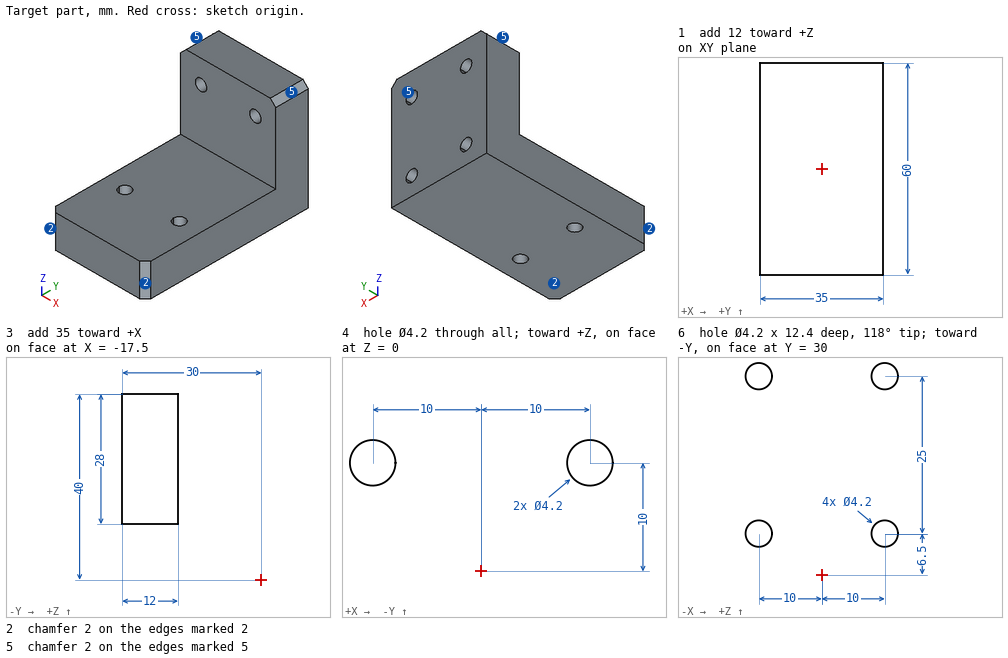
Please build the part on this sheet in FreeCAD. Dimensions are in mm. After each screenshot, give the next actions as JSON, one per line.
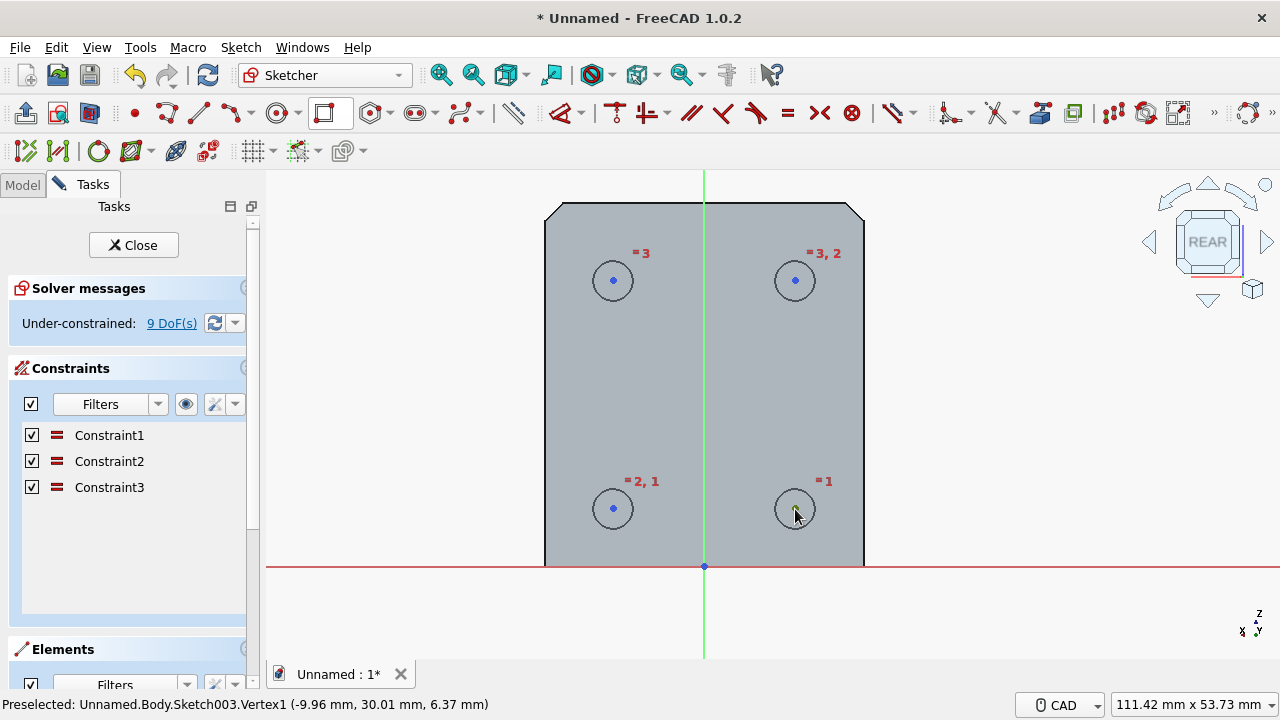
{"action": "left_click", "coordinate": [613, 509]}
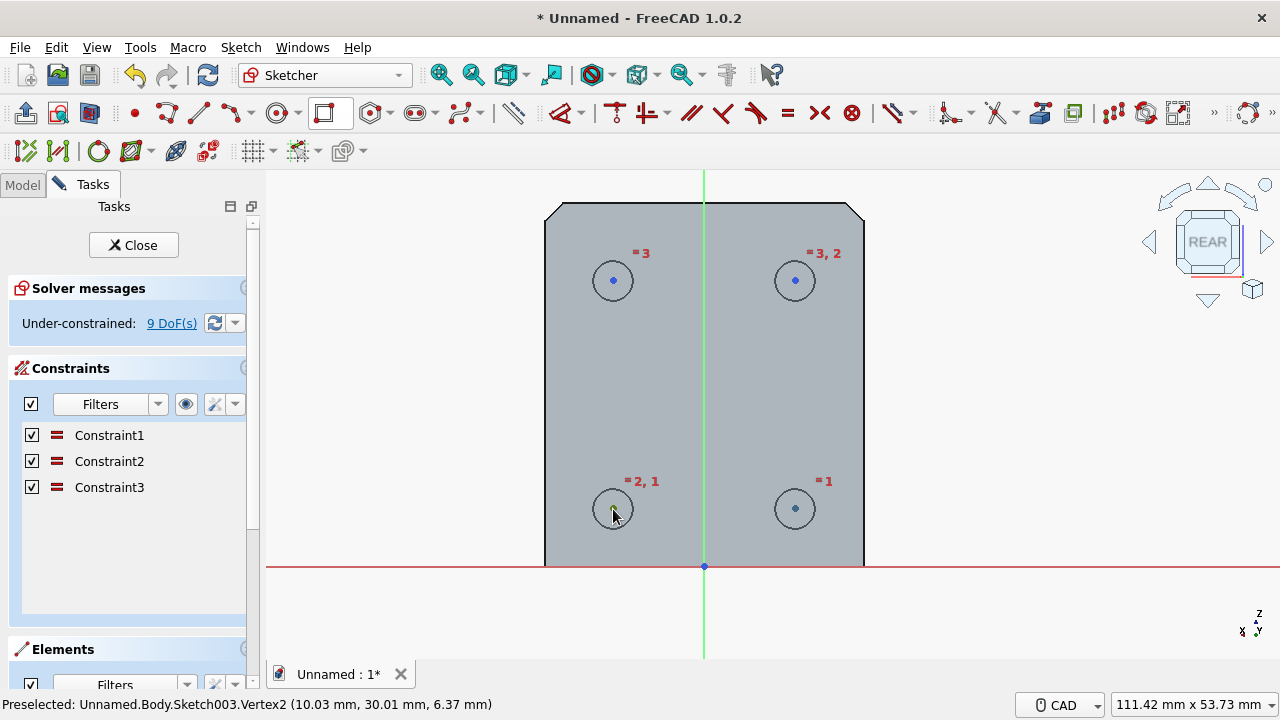
{"action": "left_click", "coordinate": [670, 114]}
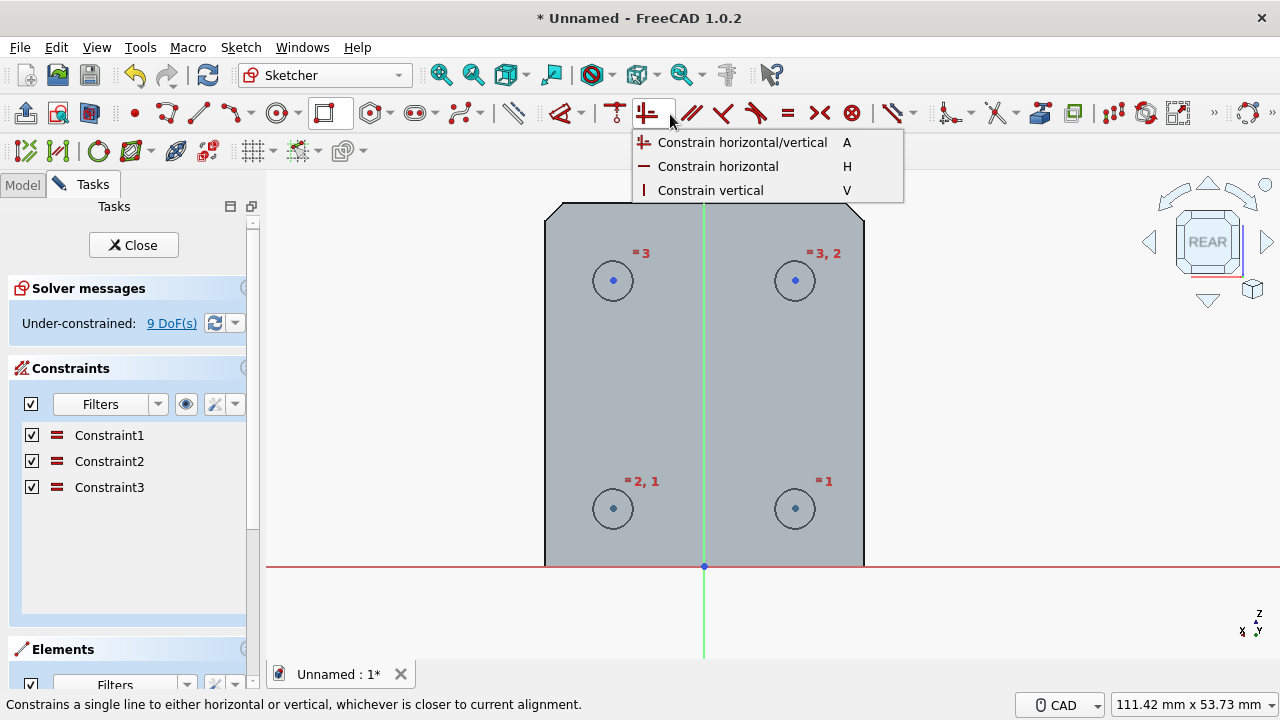
{"action": "left_click", "coordinate": [768, 166]}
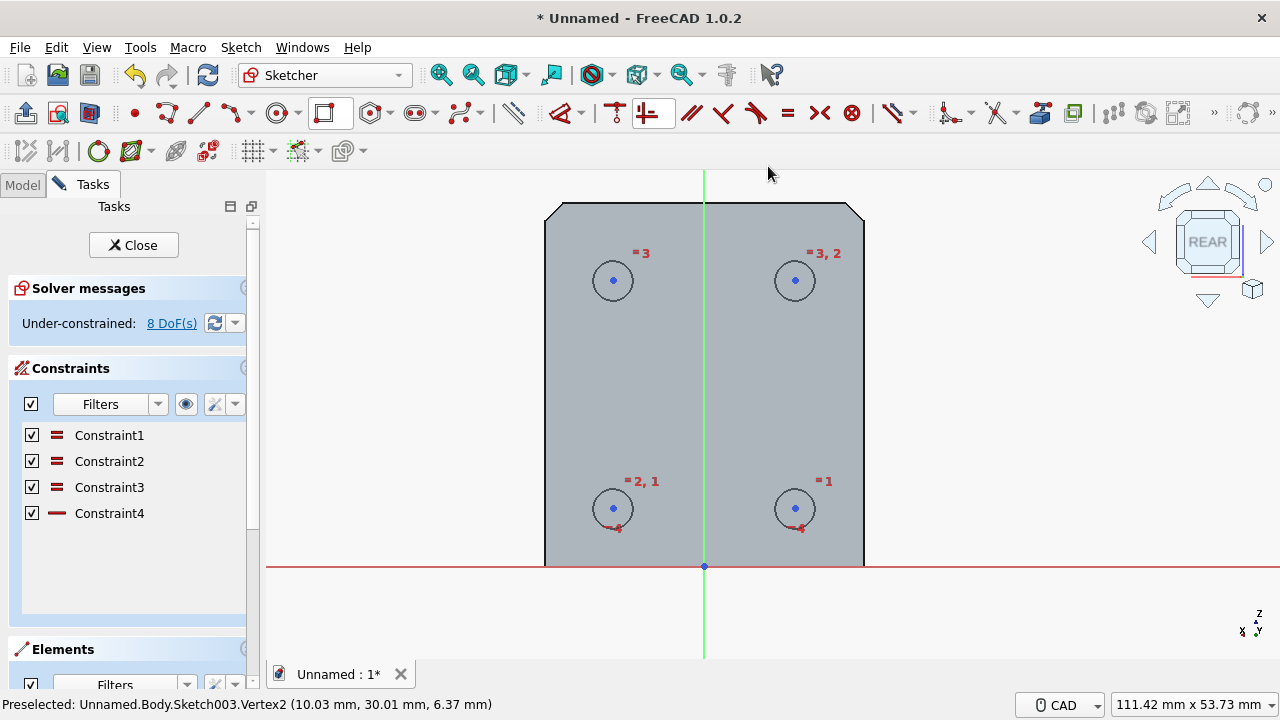
{"action": "left_click", "coordinate": [795, 509]}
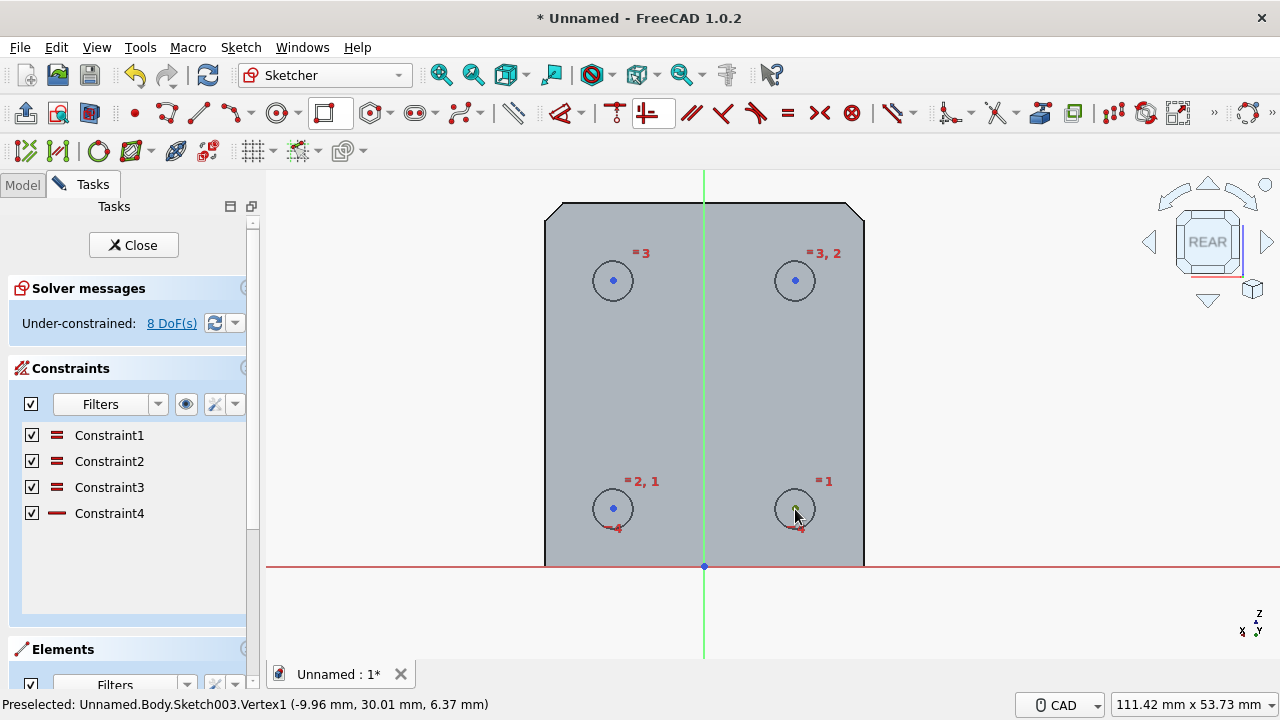
{"action": "left_click", "coordinate": [795, 281]}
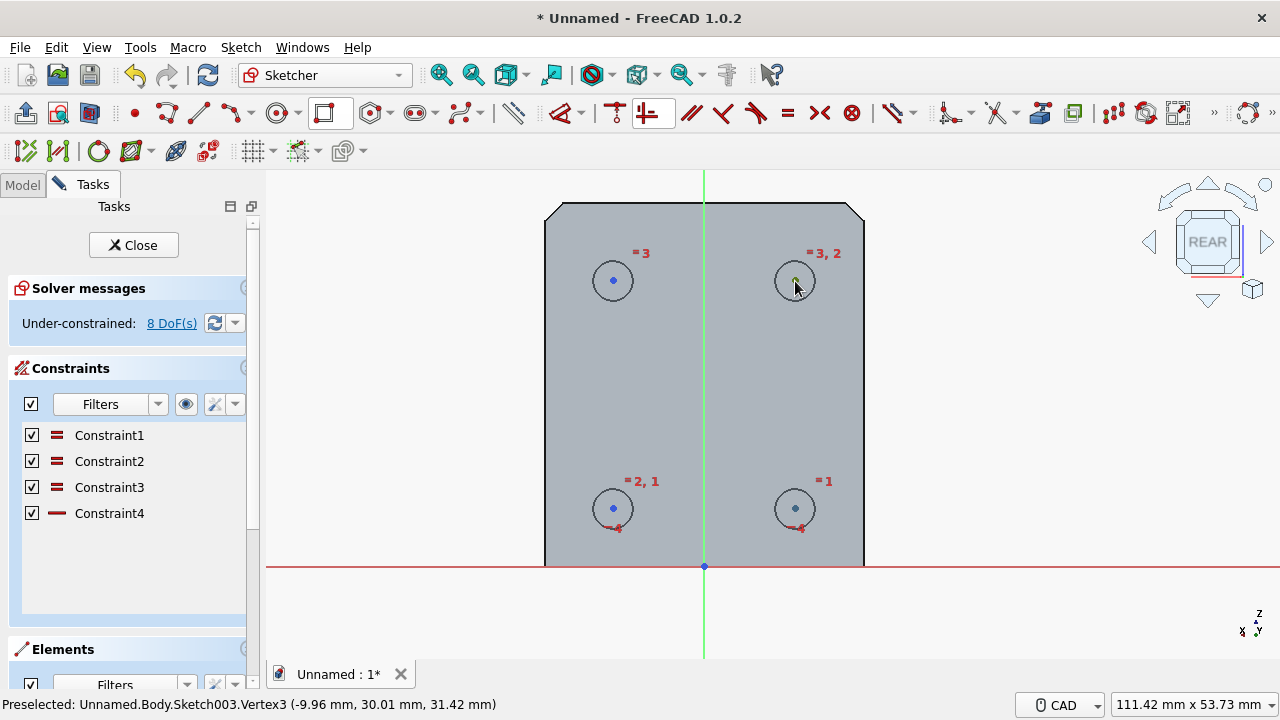
{"action": "key", "text": "v"}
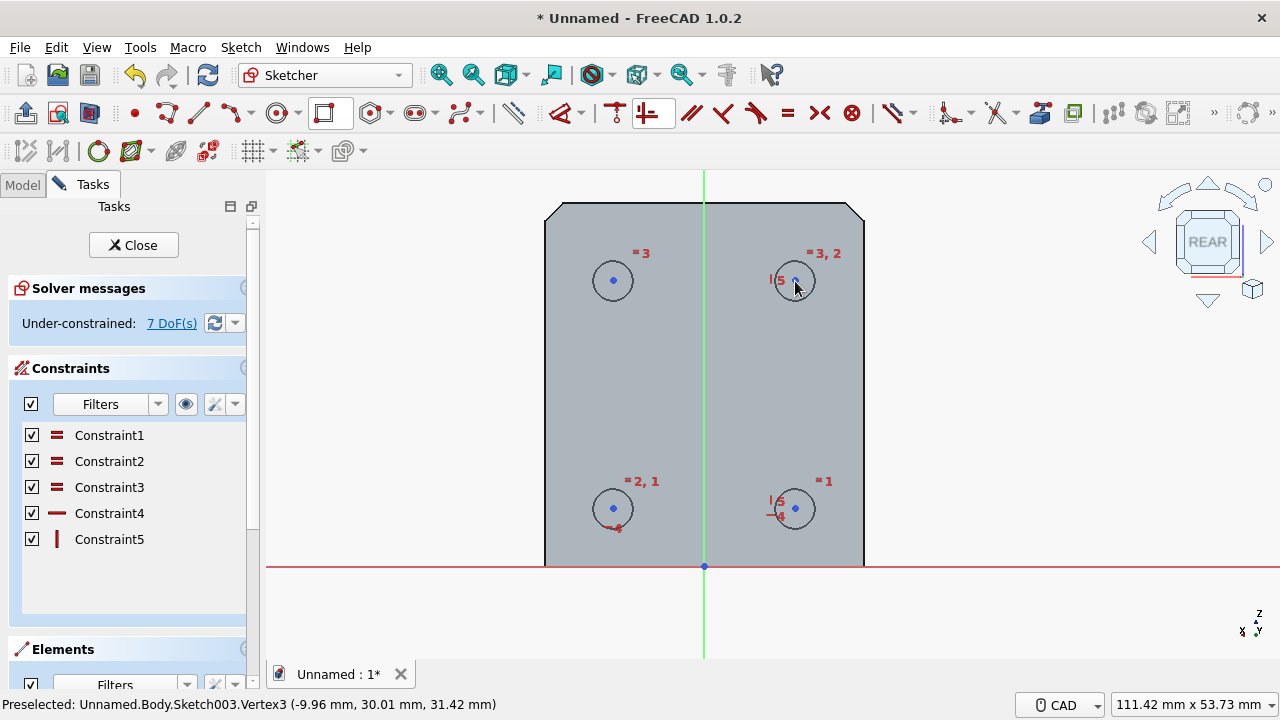
{"action": "left_click", "coordinate": [613, 509]}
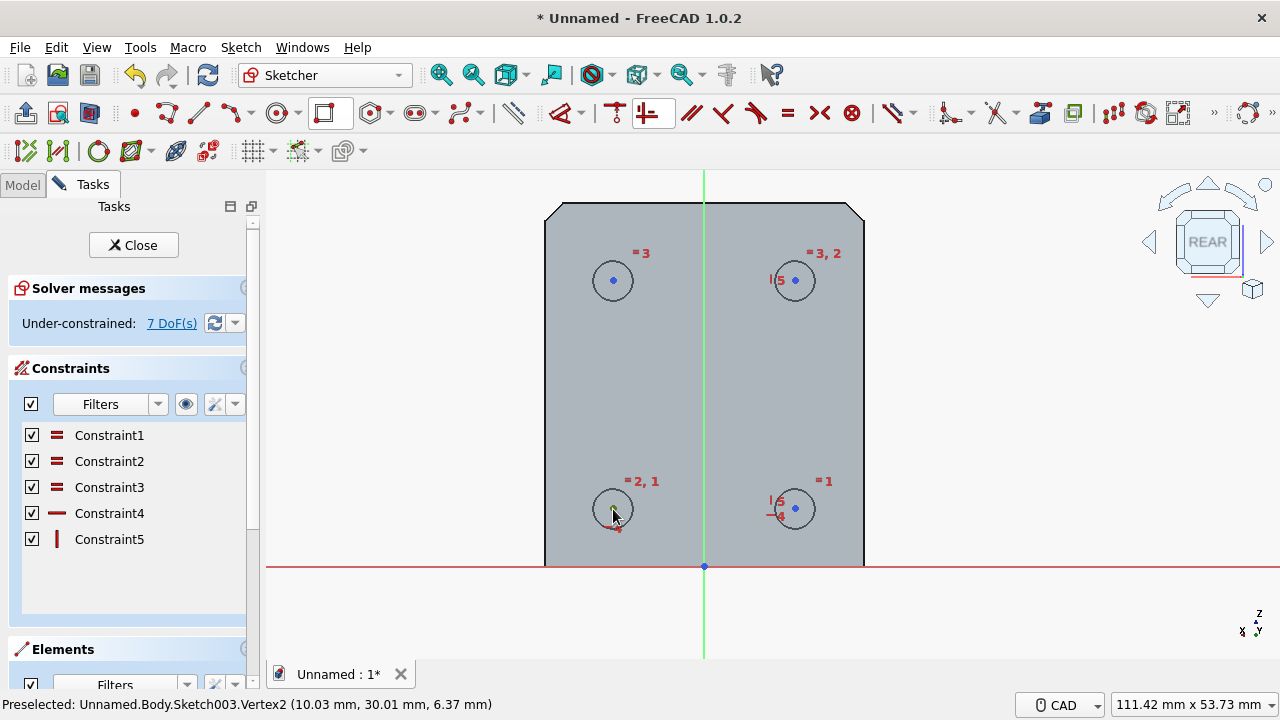
{"action": "left_click", "coordinate": [613, 281]}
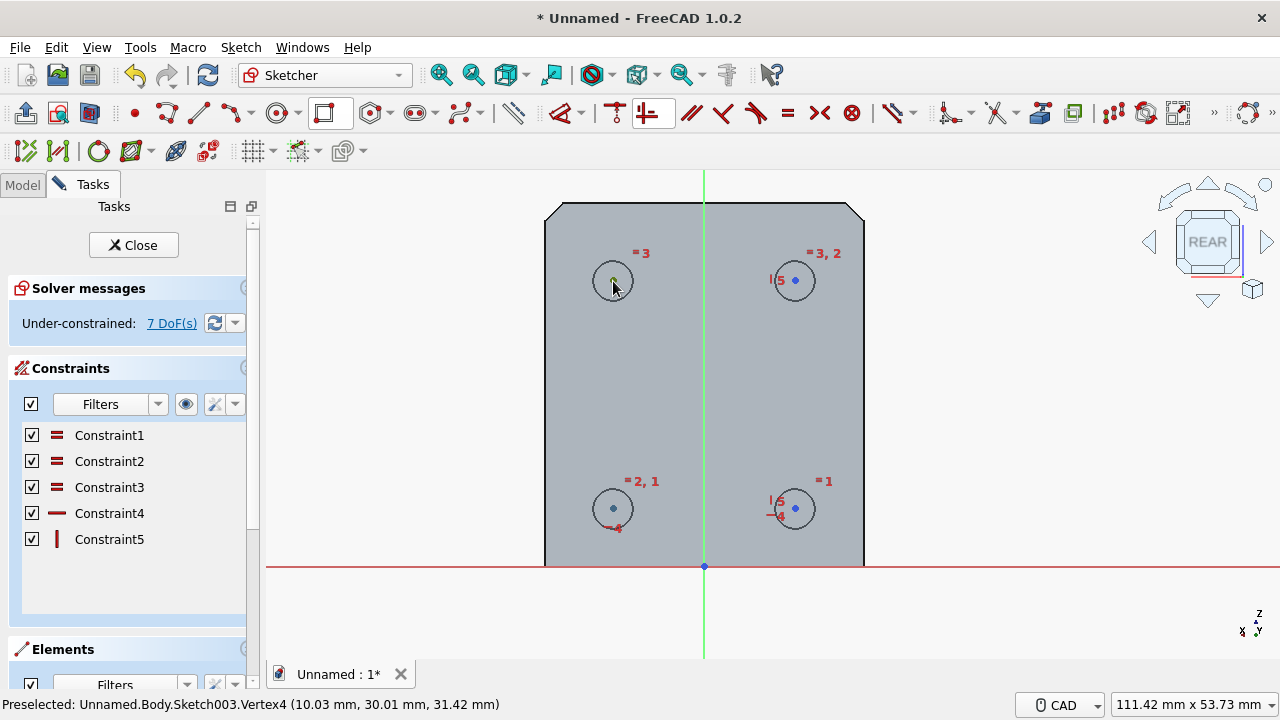
{"action": "left_click", "coordinate": [670, 114]}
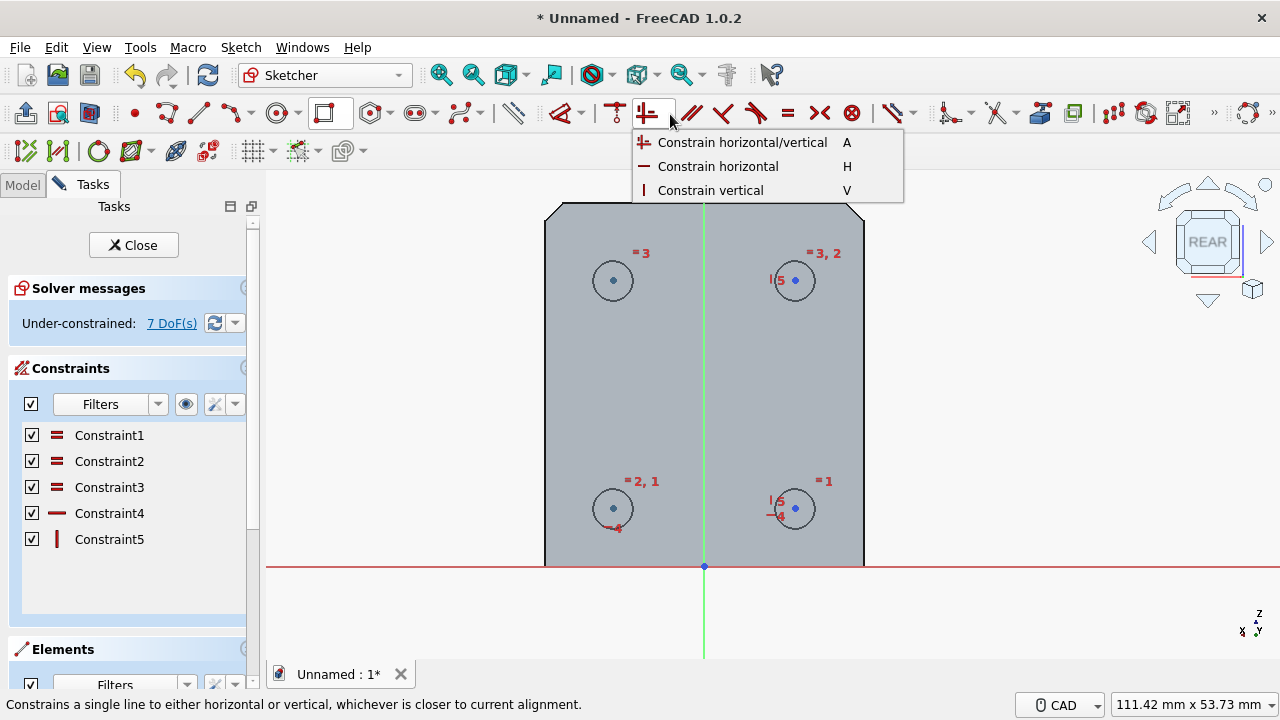
{"action": "left_click", "coordinate": [768, 190]}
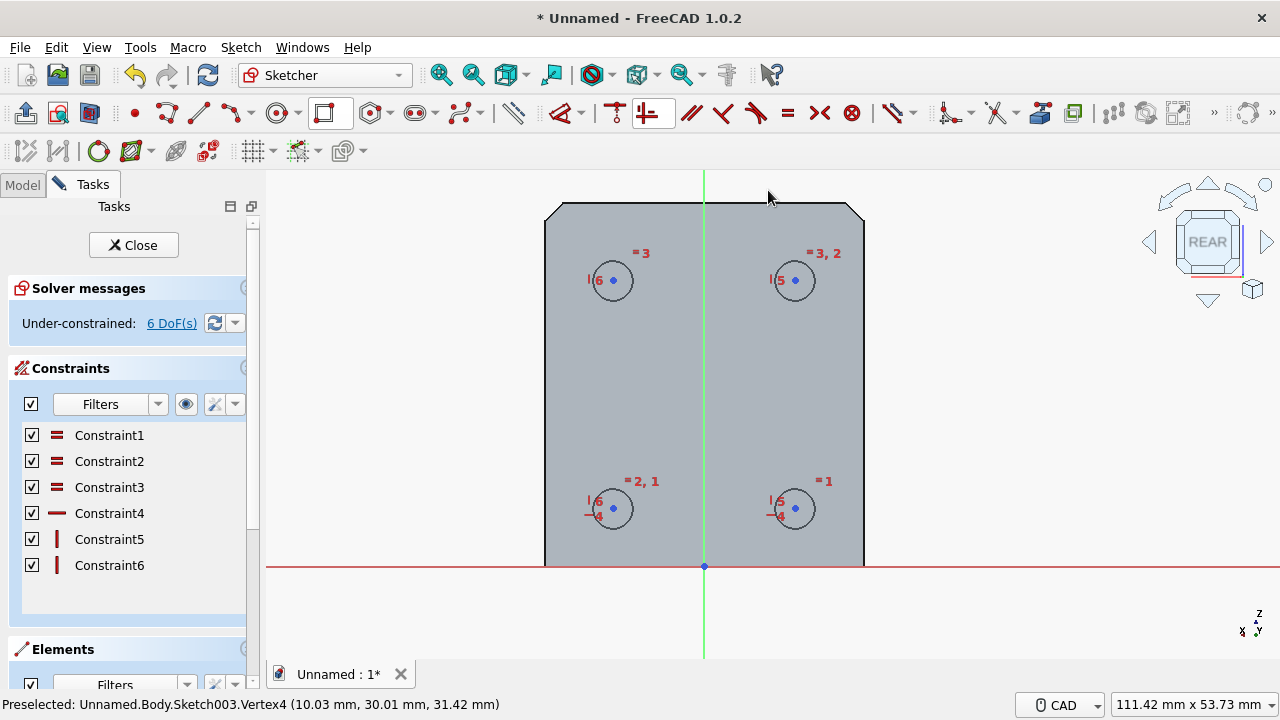
{"action": "left_click", "coordinate": [795, 281]}